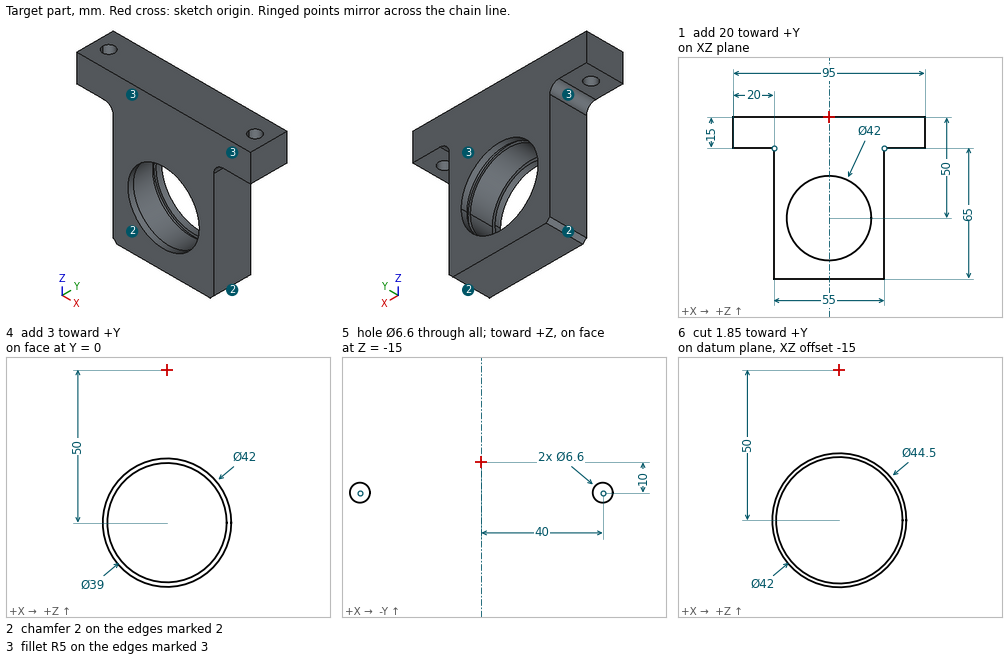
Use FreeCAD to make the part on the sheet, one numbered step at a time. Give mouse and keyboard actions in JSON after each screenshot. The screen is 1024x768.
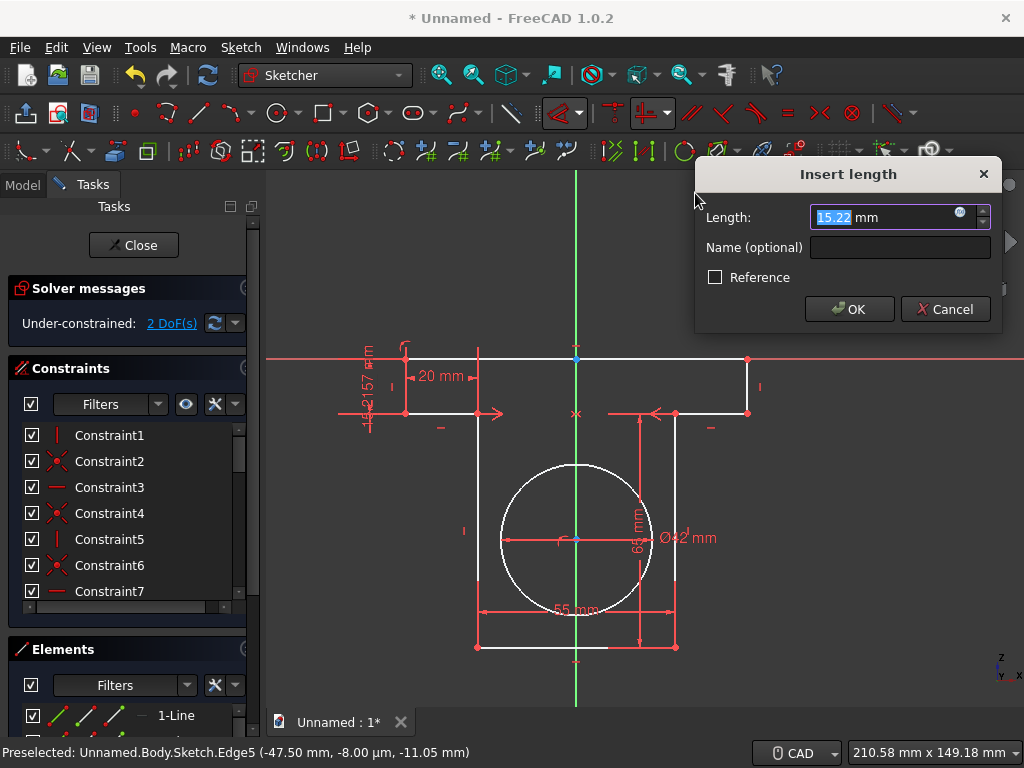
{"action": "type", "text": "15"}
{"action": "key", "text": "Return"}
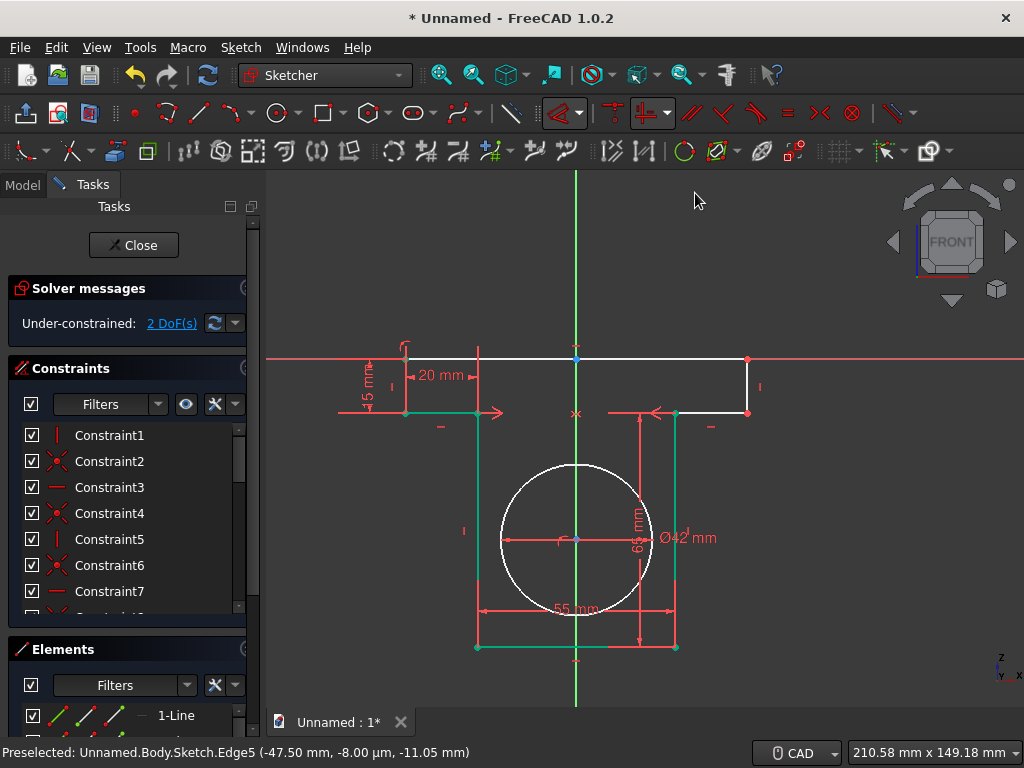
{"action": "left_click", "coordinate": [508, 359]}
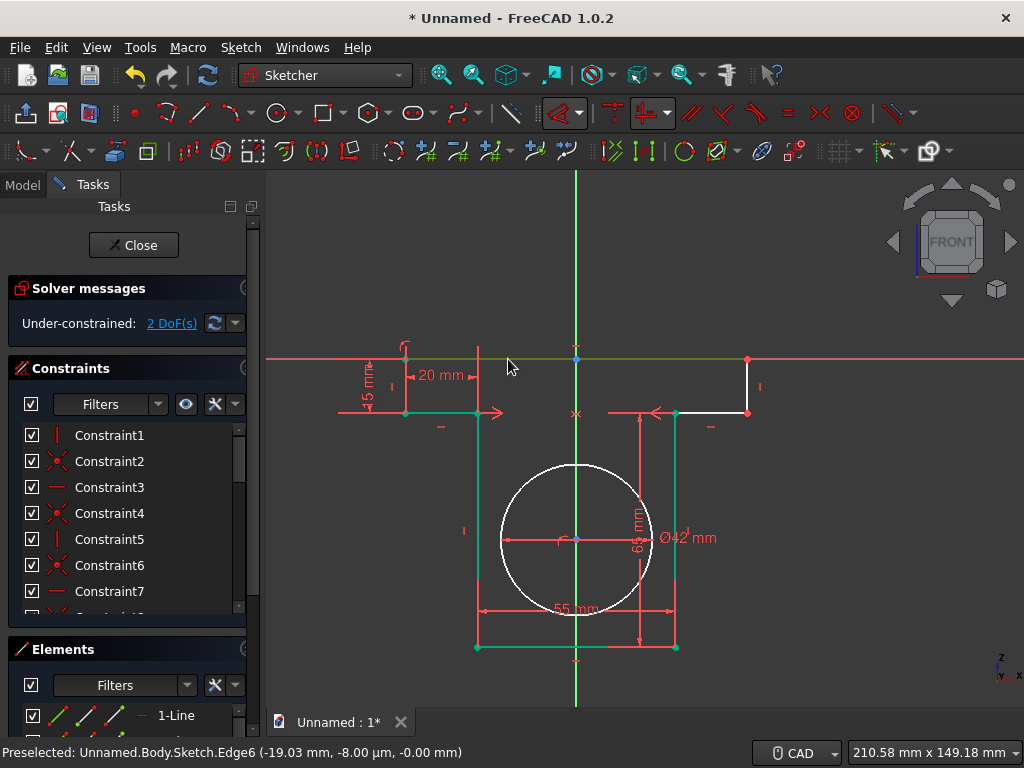
{"action": "left_click", "coordinate": [582, 114]}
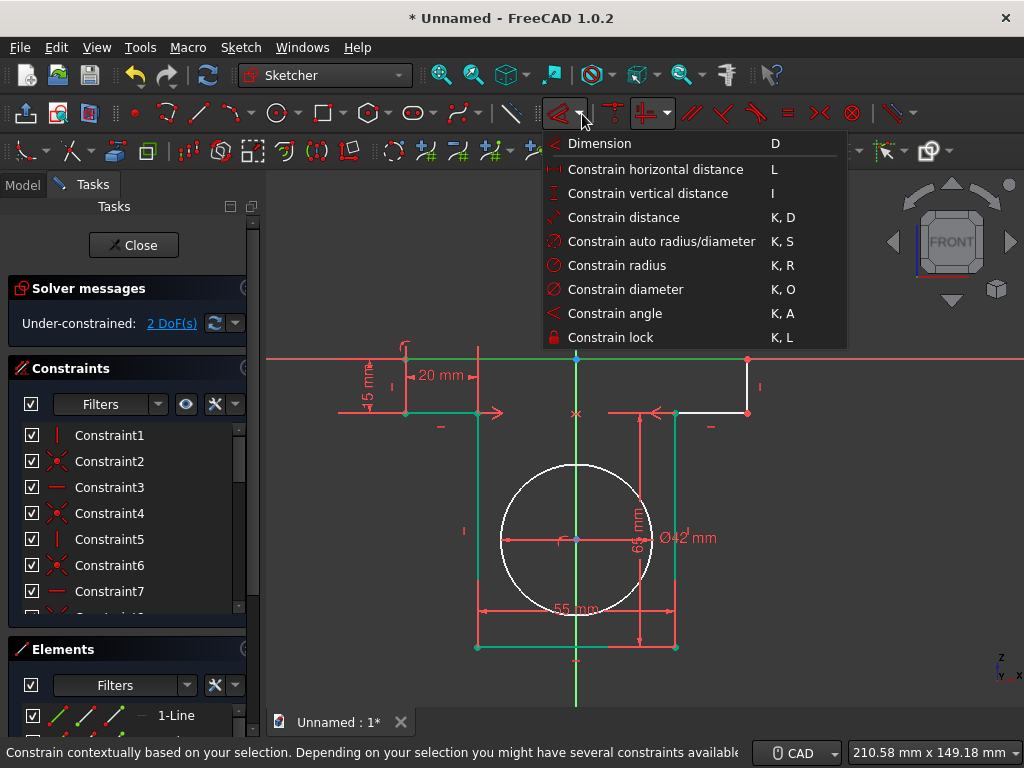
{"action": "left_click", "coordinate": [695, 169]}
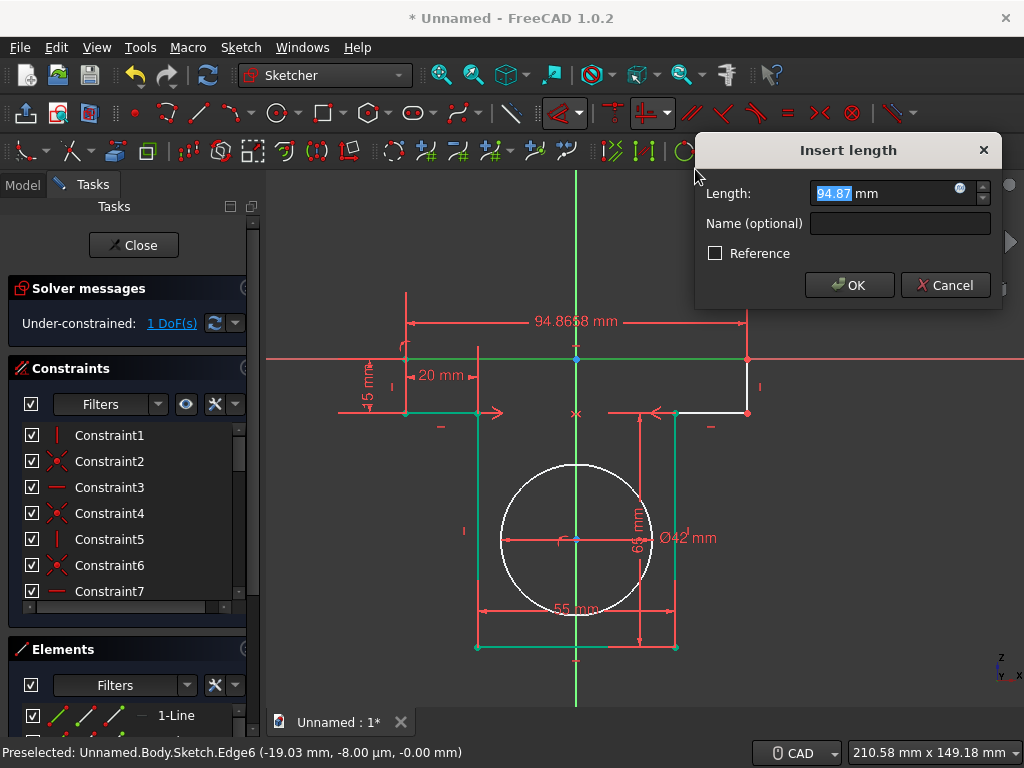
{"action": "type", "text": "95"}
{"action": "key", "text": "Return"}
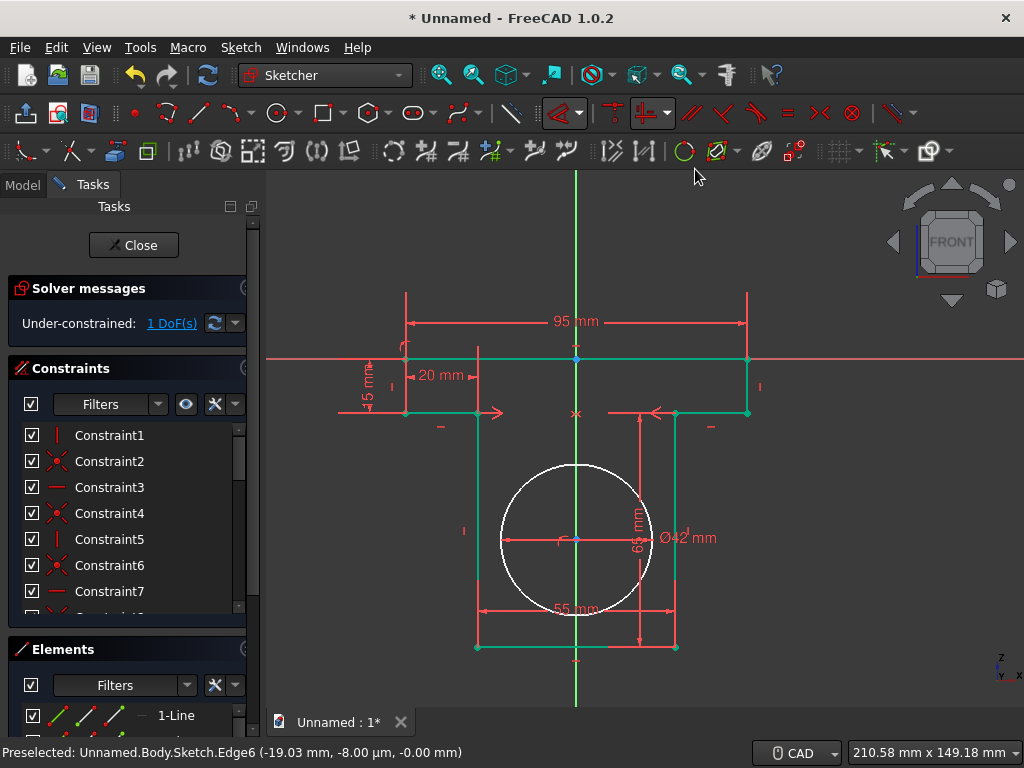
{"action": "left_click", "coordinate": [577, 540]}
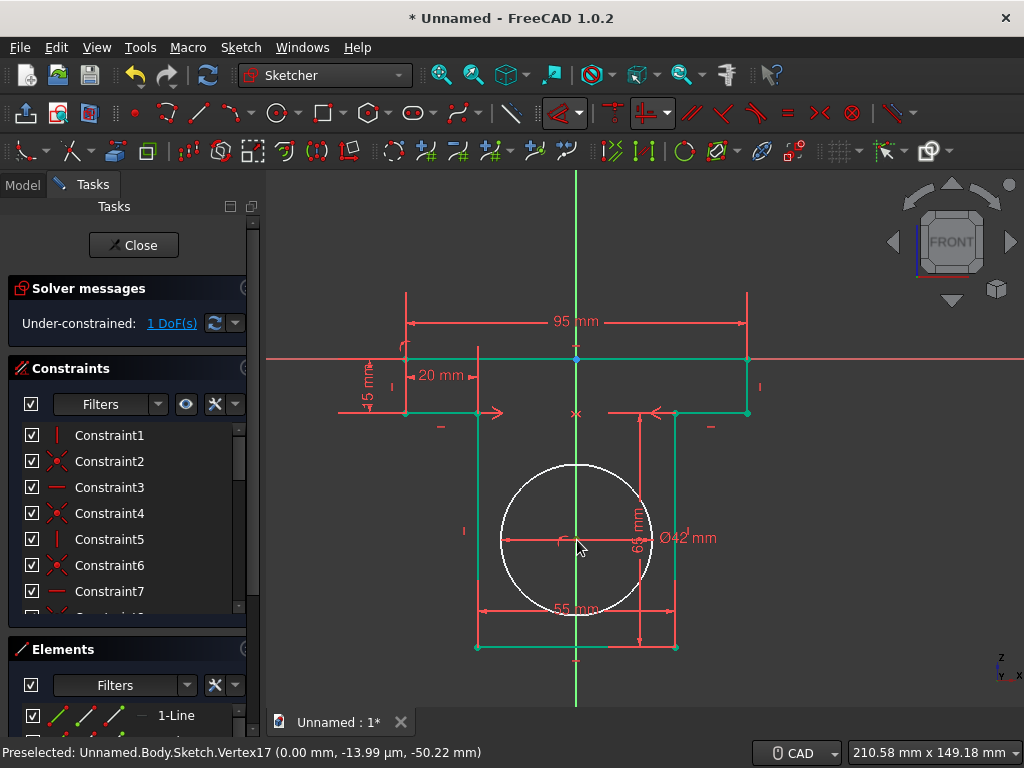
{"action": "key", "text": "i"}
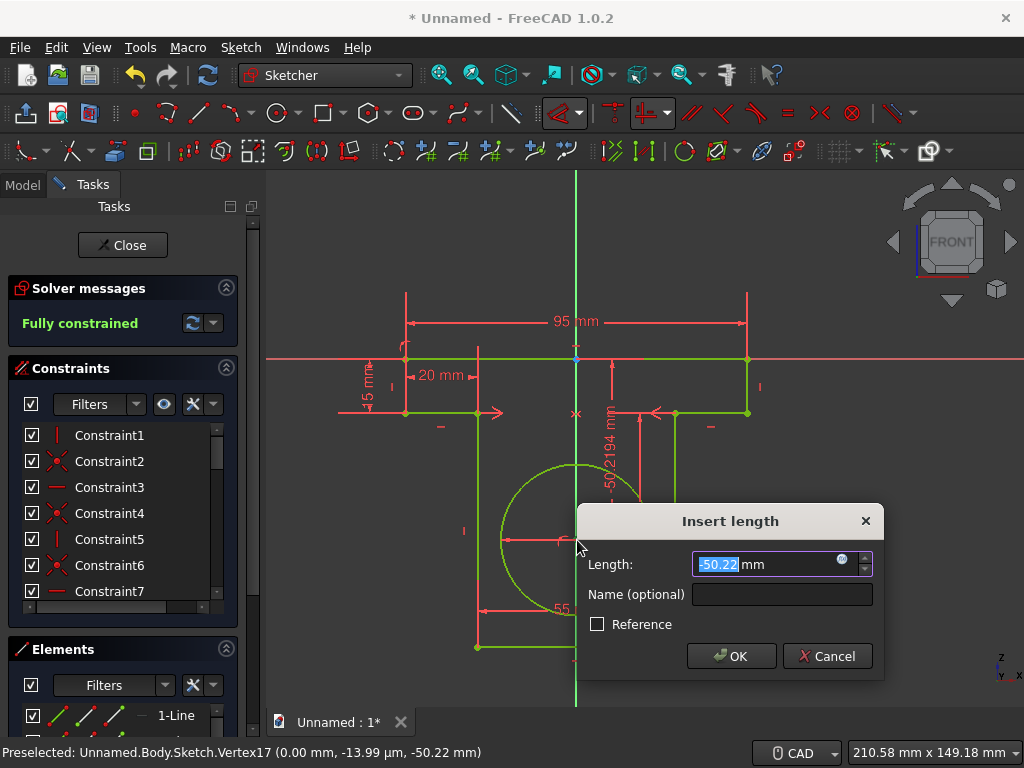
{"action": "type", "text": "-50"}
{"action": "key", "text": "Return"}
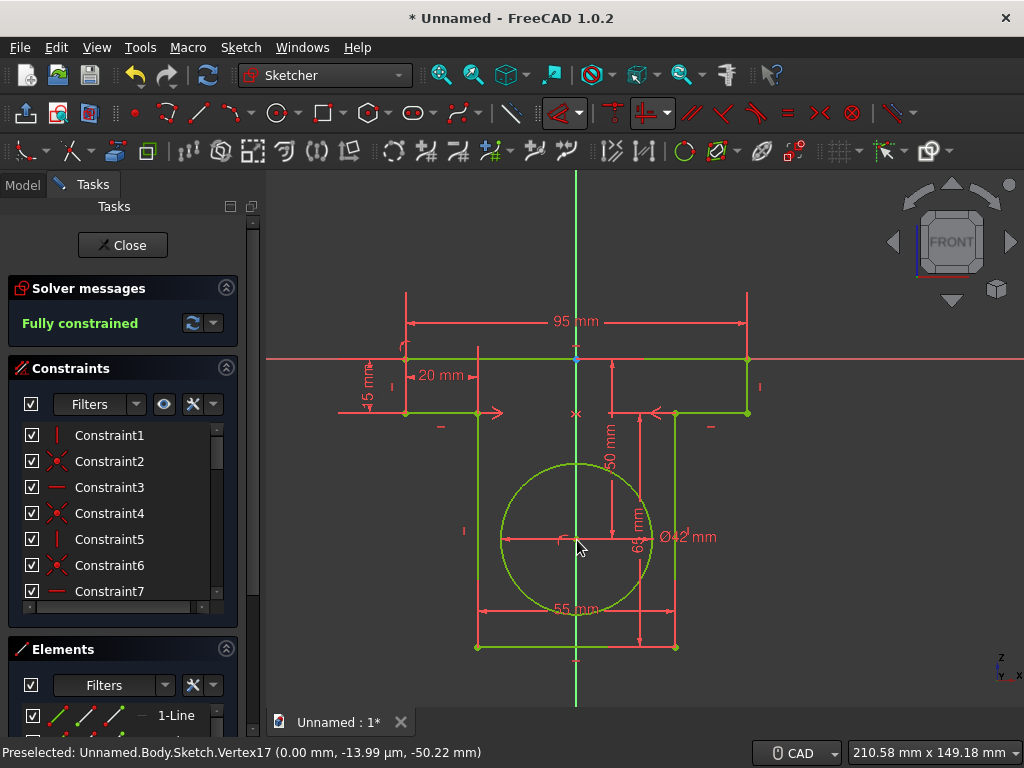
{"action": "left_click", "coordinate": [123, 245]}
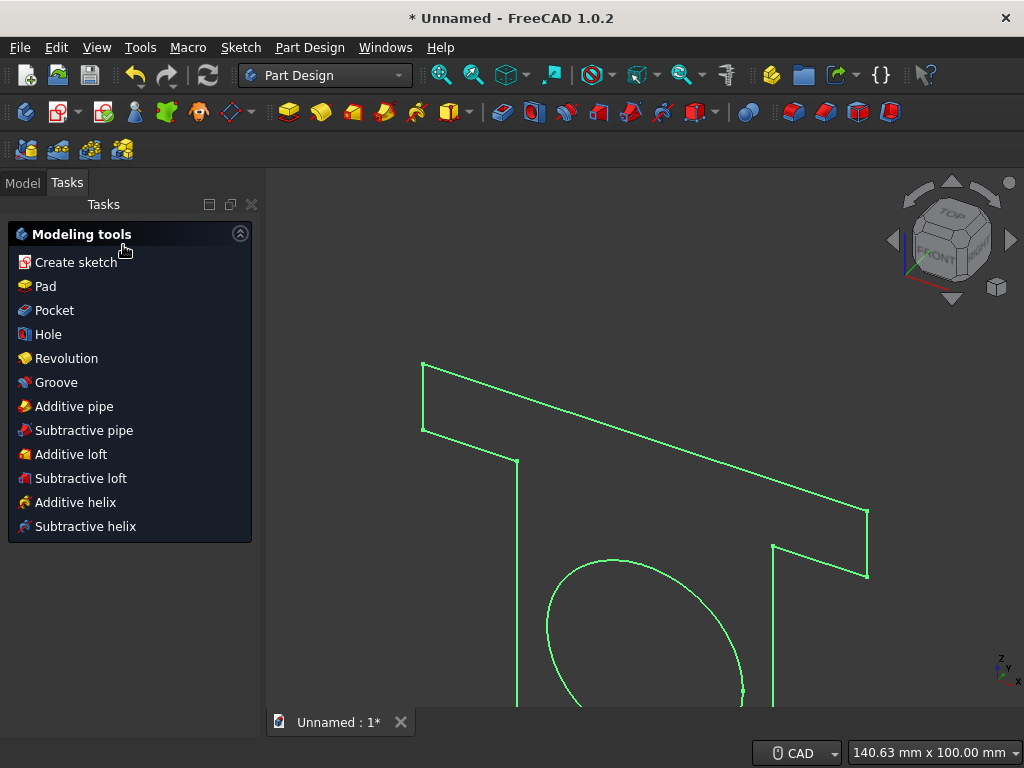
{"action": "left_click", "coordinate": [290, 112]}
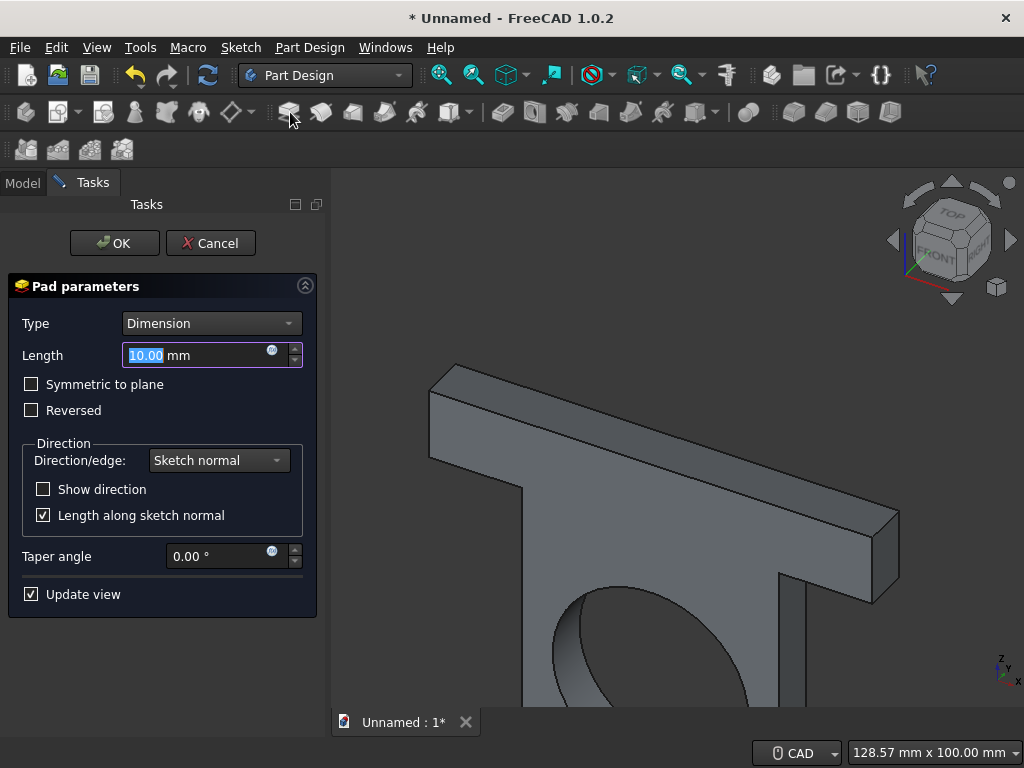
{"action": "type", "text": "20"}
{"action": "key", "text": "Tab"}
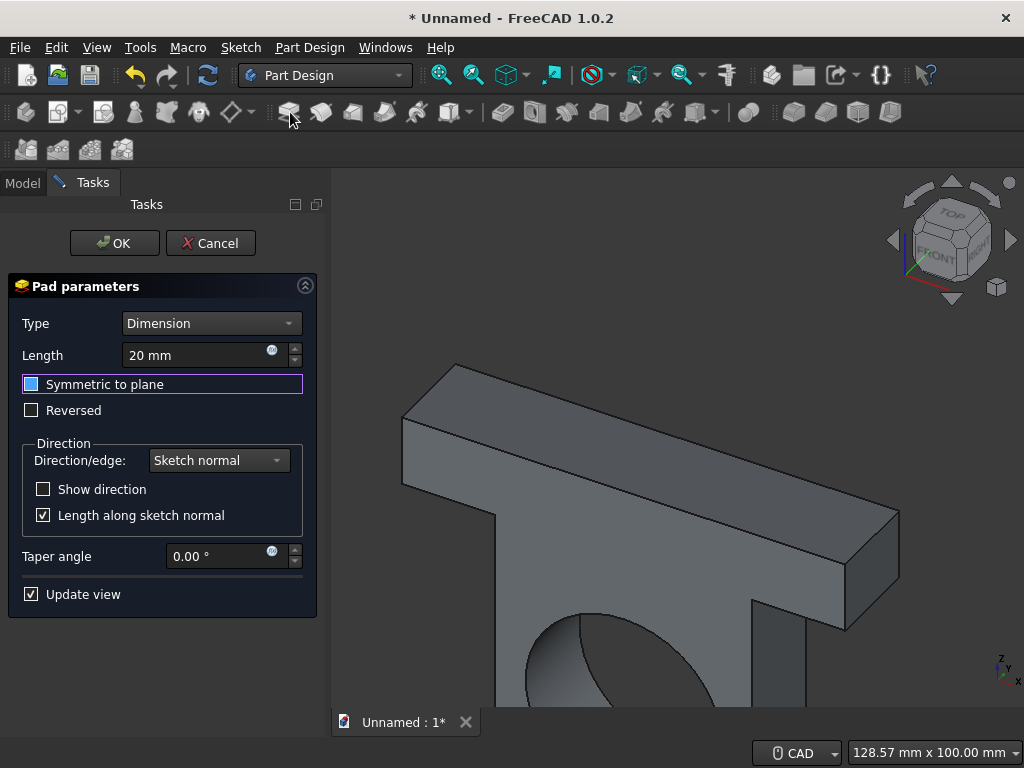
{"action": "left_click", "coordinate": [30, 410]}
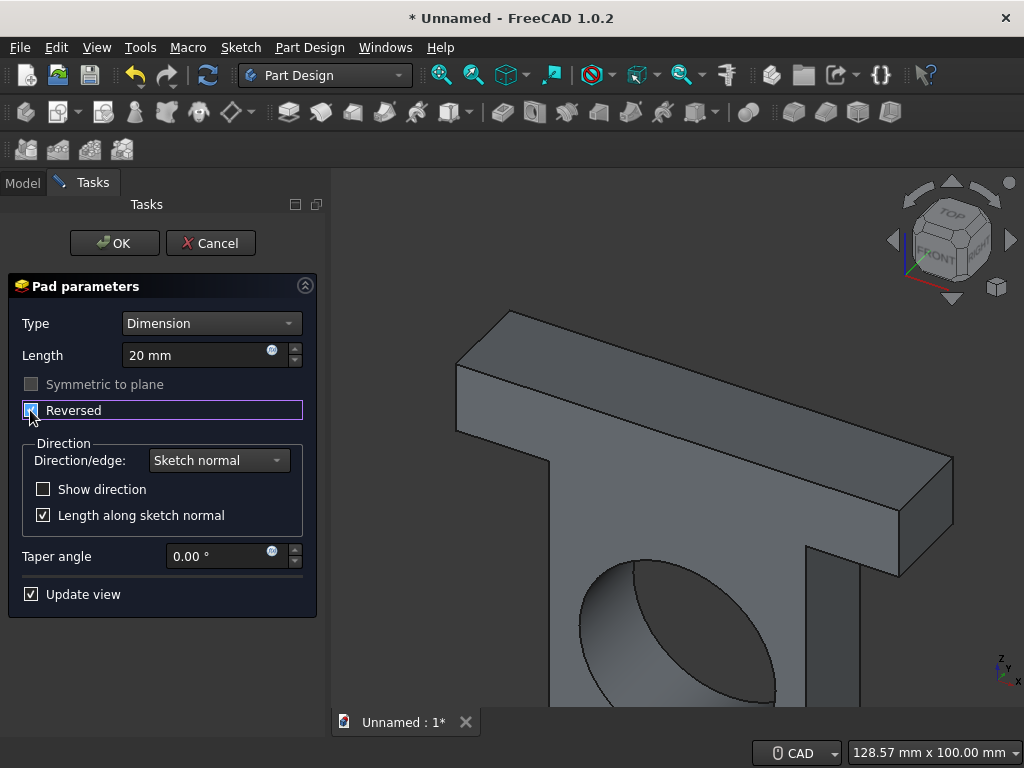
{"action": "left_click", "coordinate": [115, 243]}